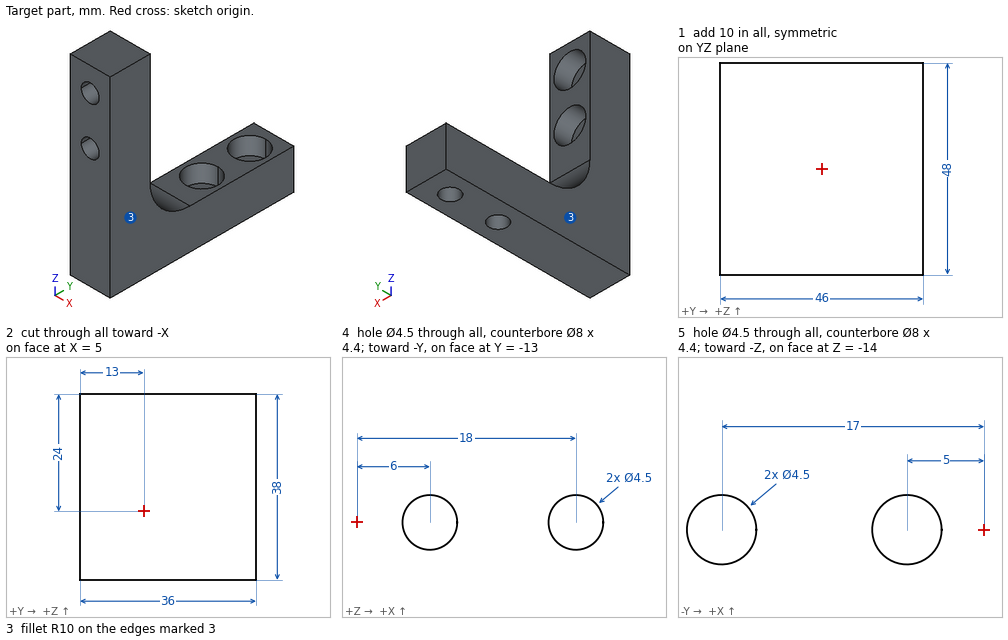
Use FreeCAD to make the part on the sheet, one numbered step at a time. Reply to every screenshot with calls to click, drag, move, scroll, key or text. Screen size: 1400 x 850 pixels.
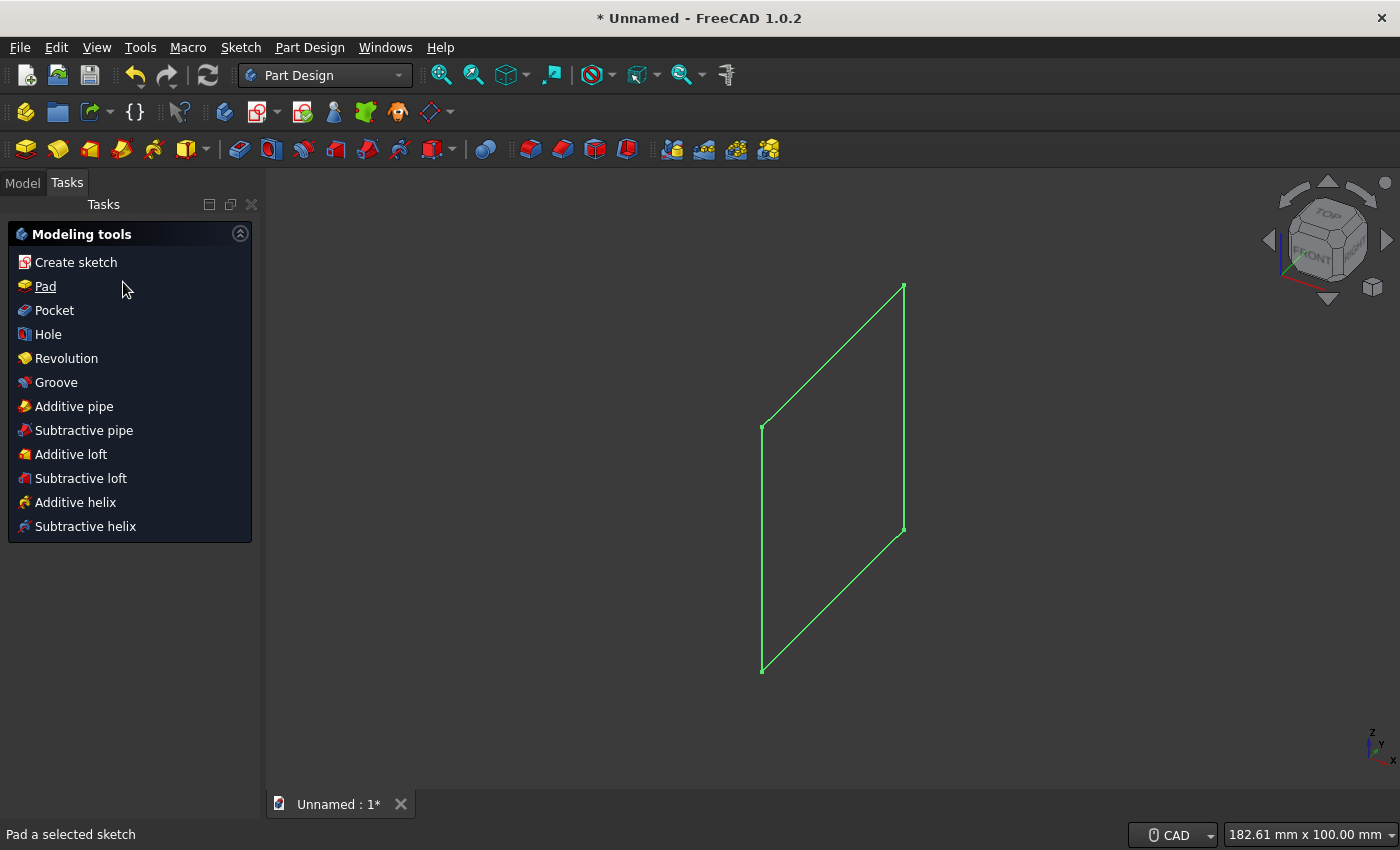
click(26, 150)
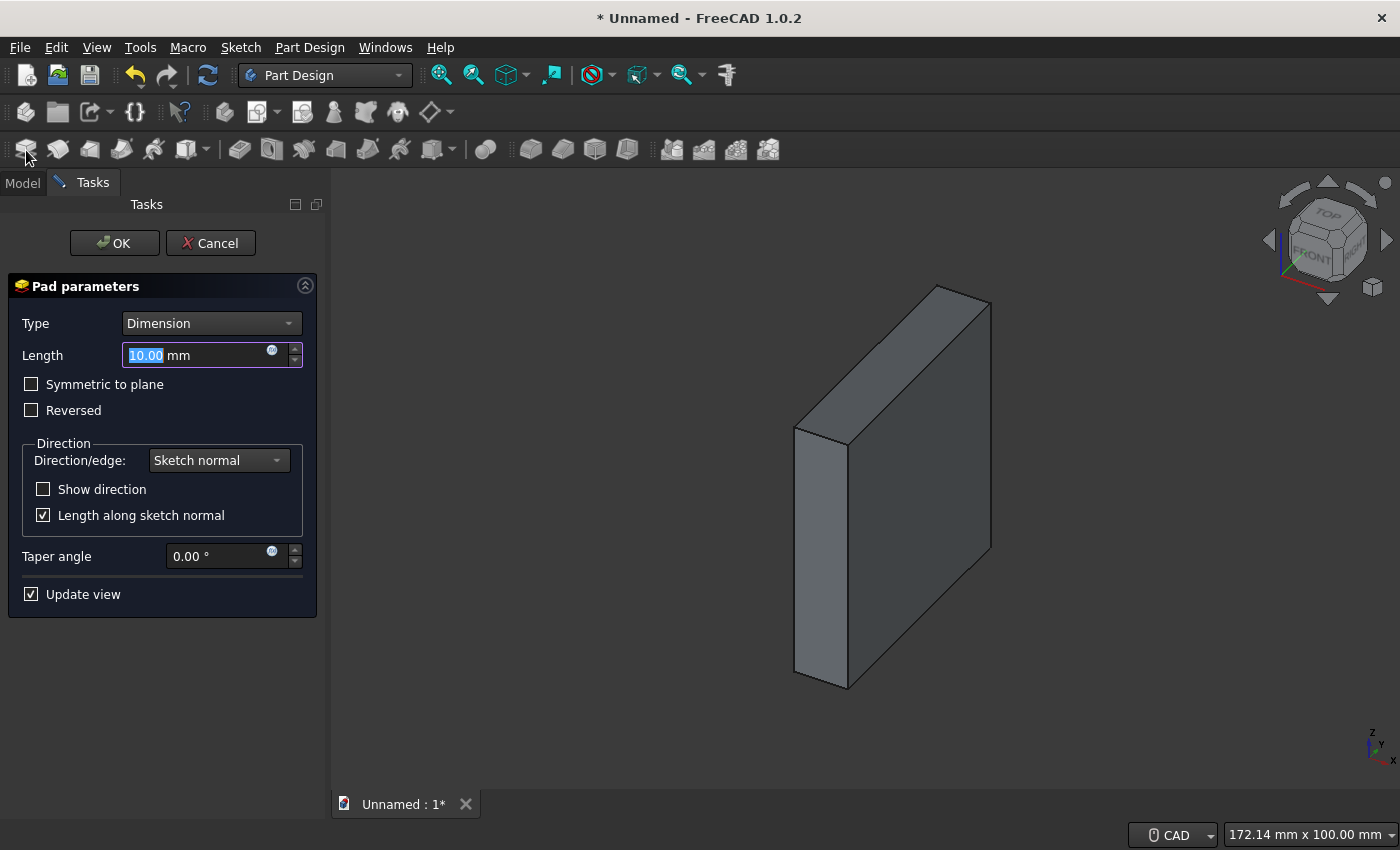
text(10)
key(Tab)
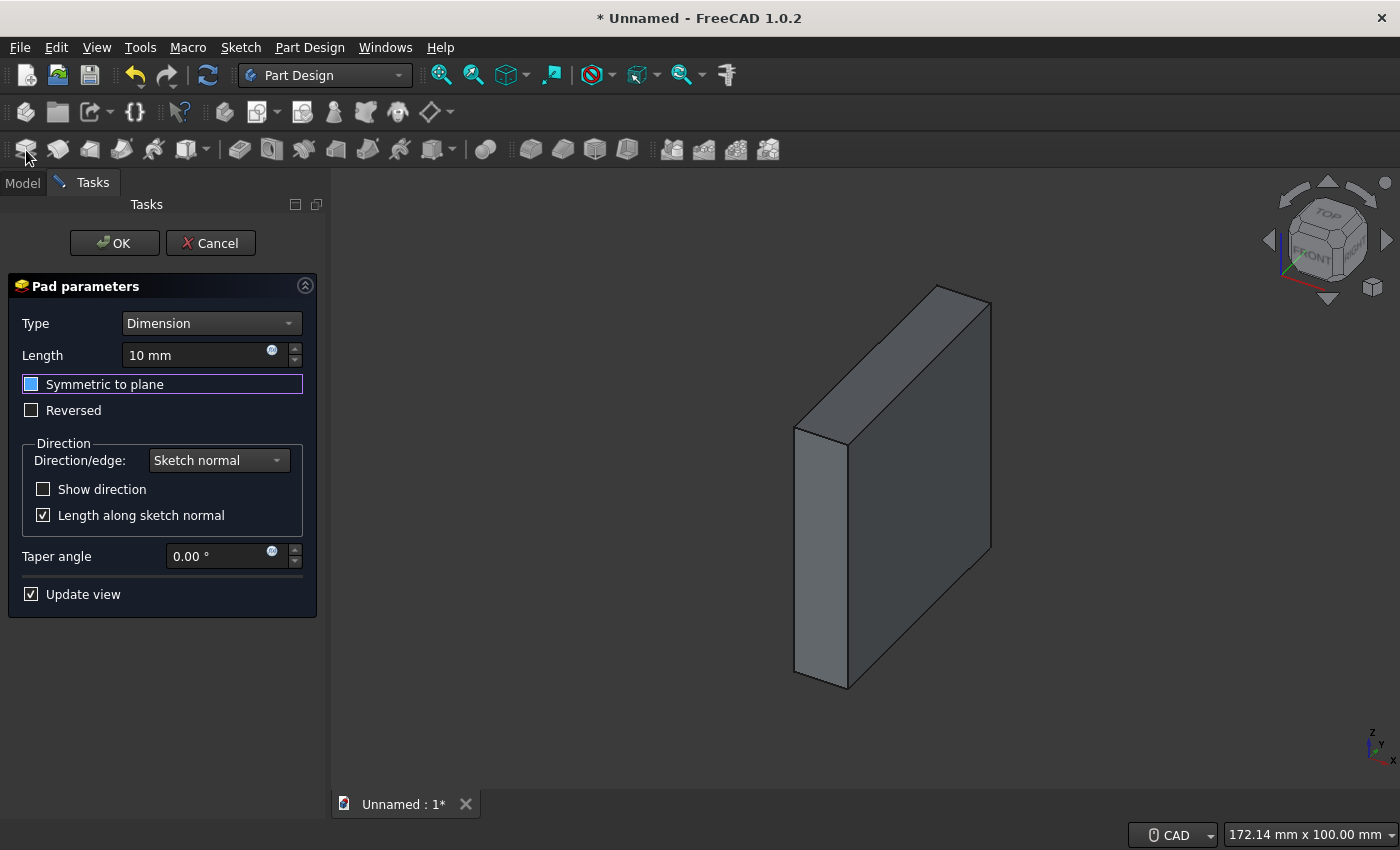
click(30, 384)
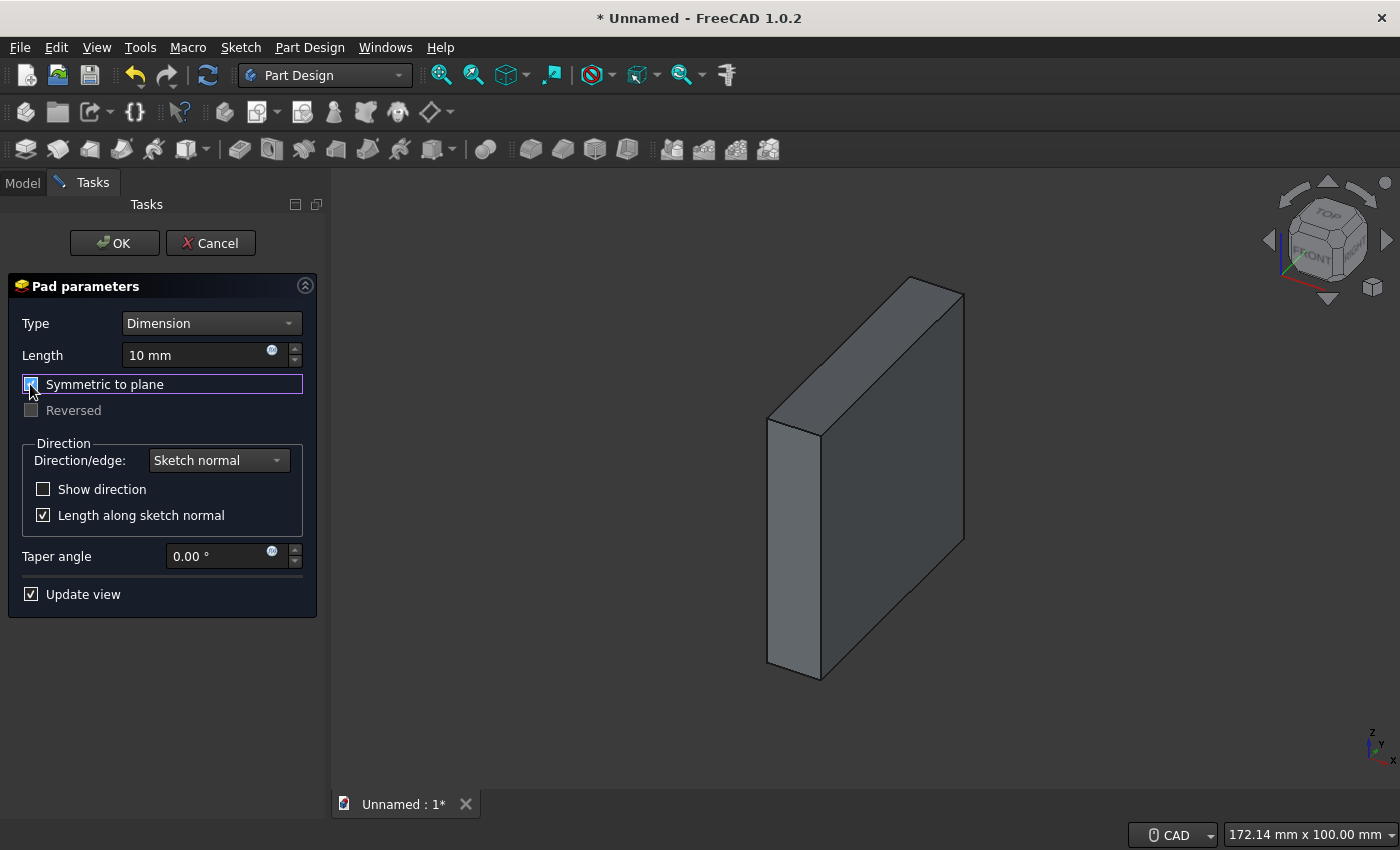
click(115, 243)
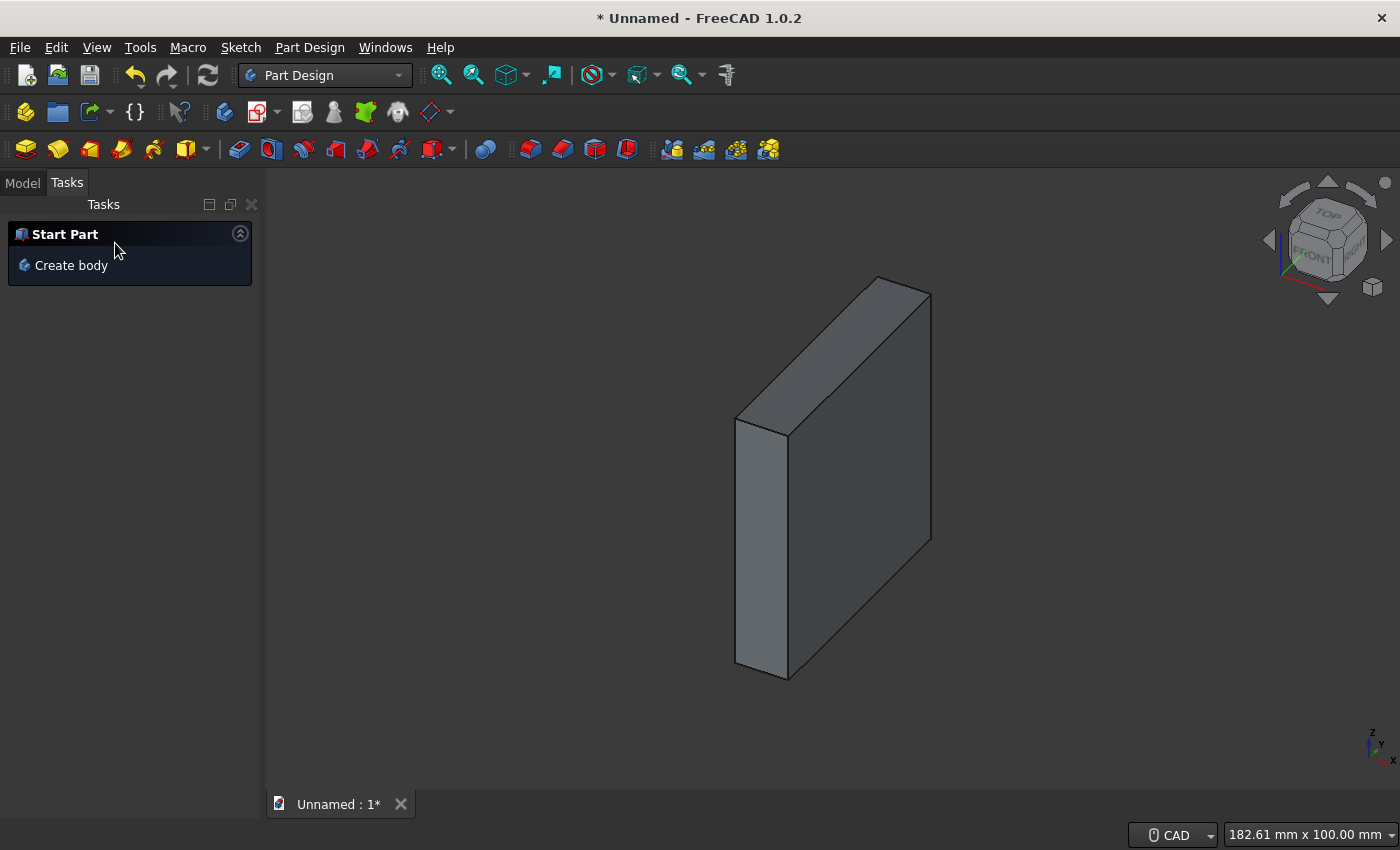
click(860, 486)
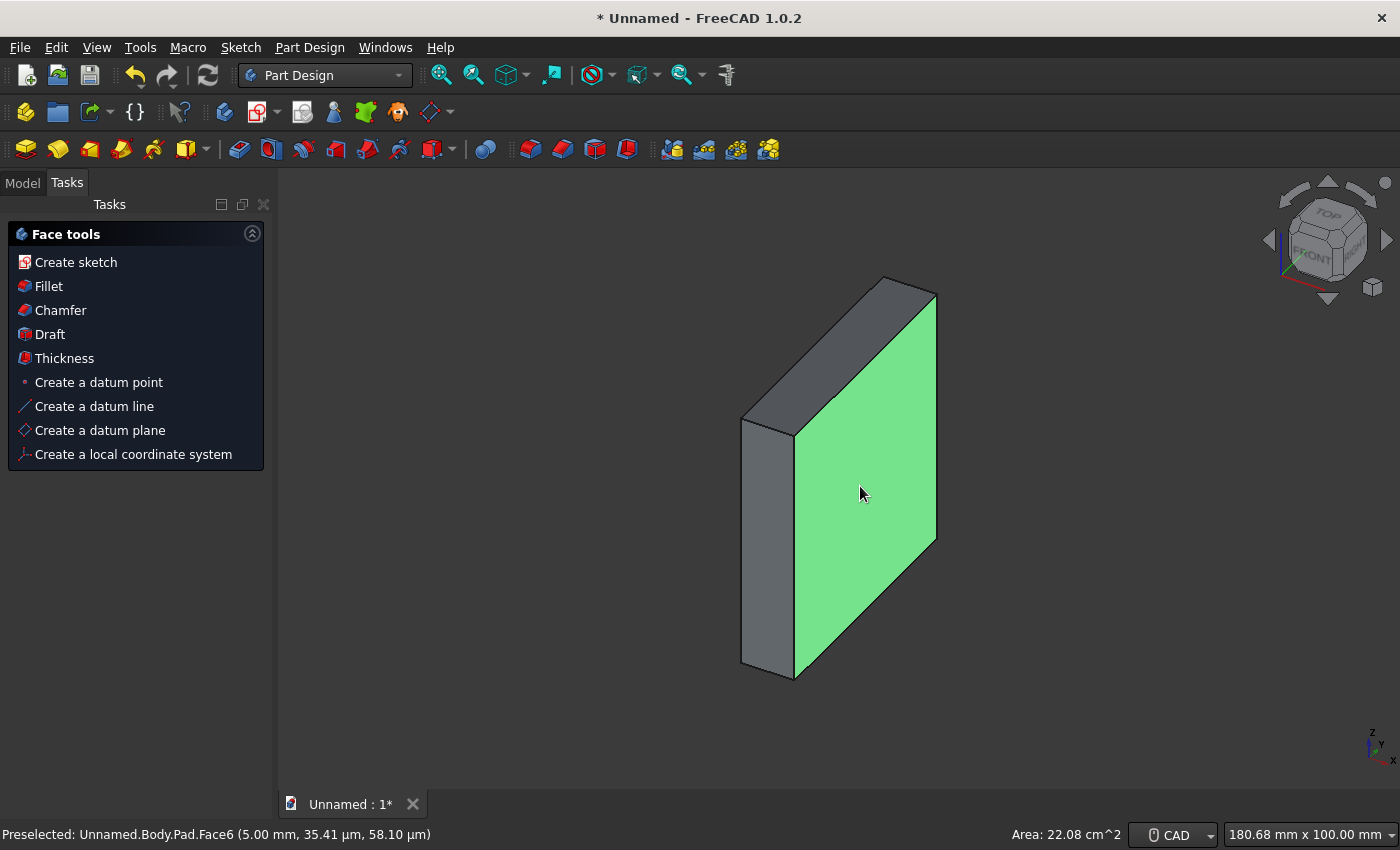
click(258, 112)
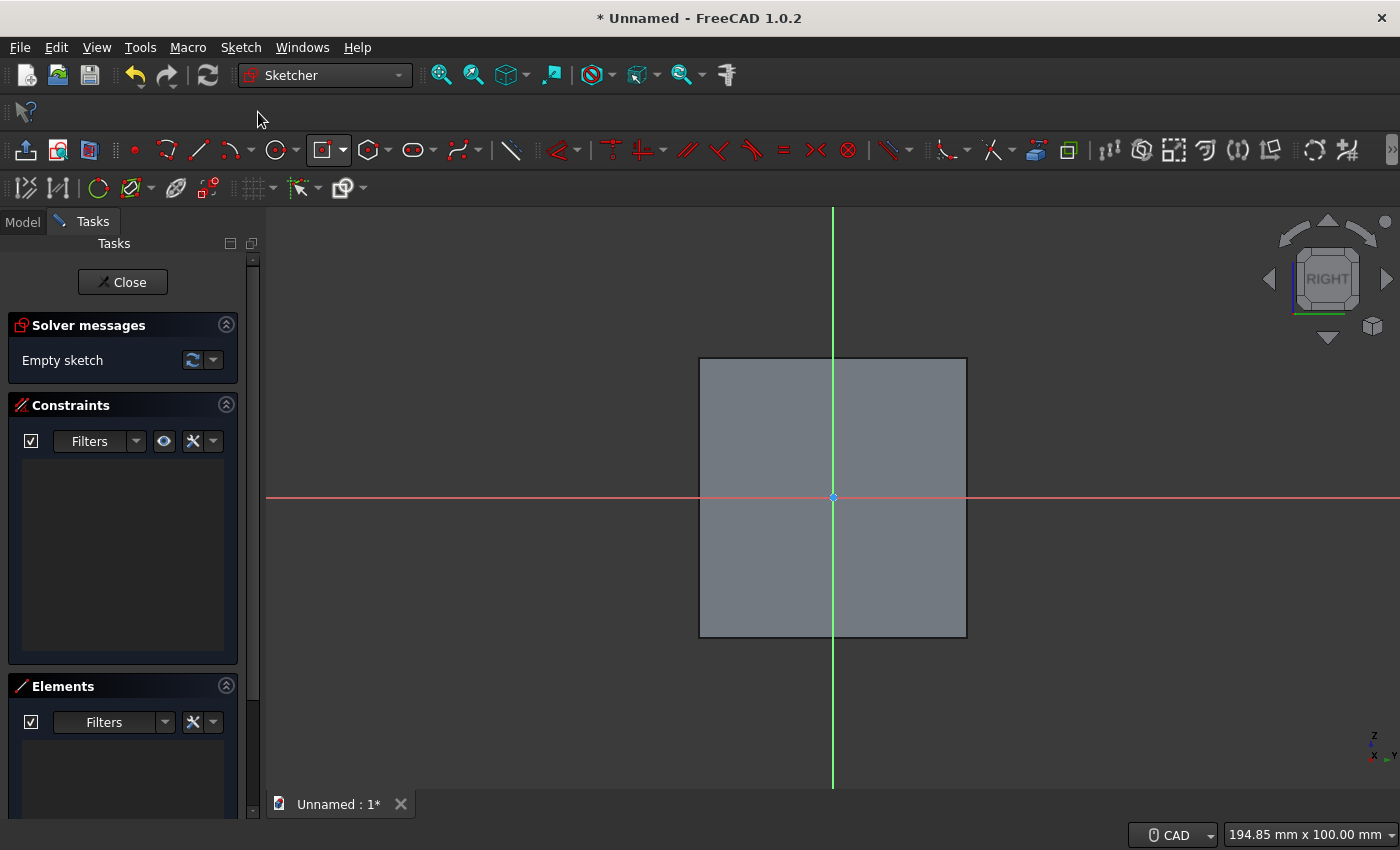
scroll(981, 434, up, 3)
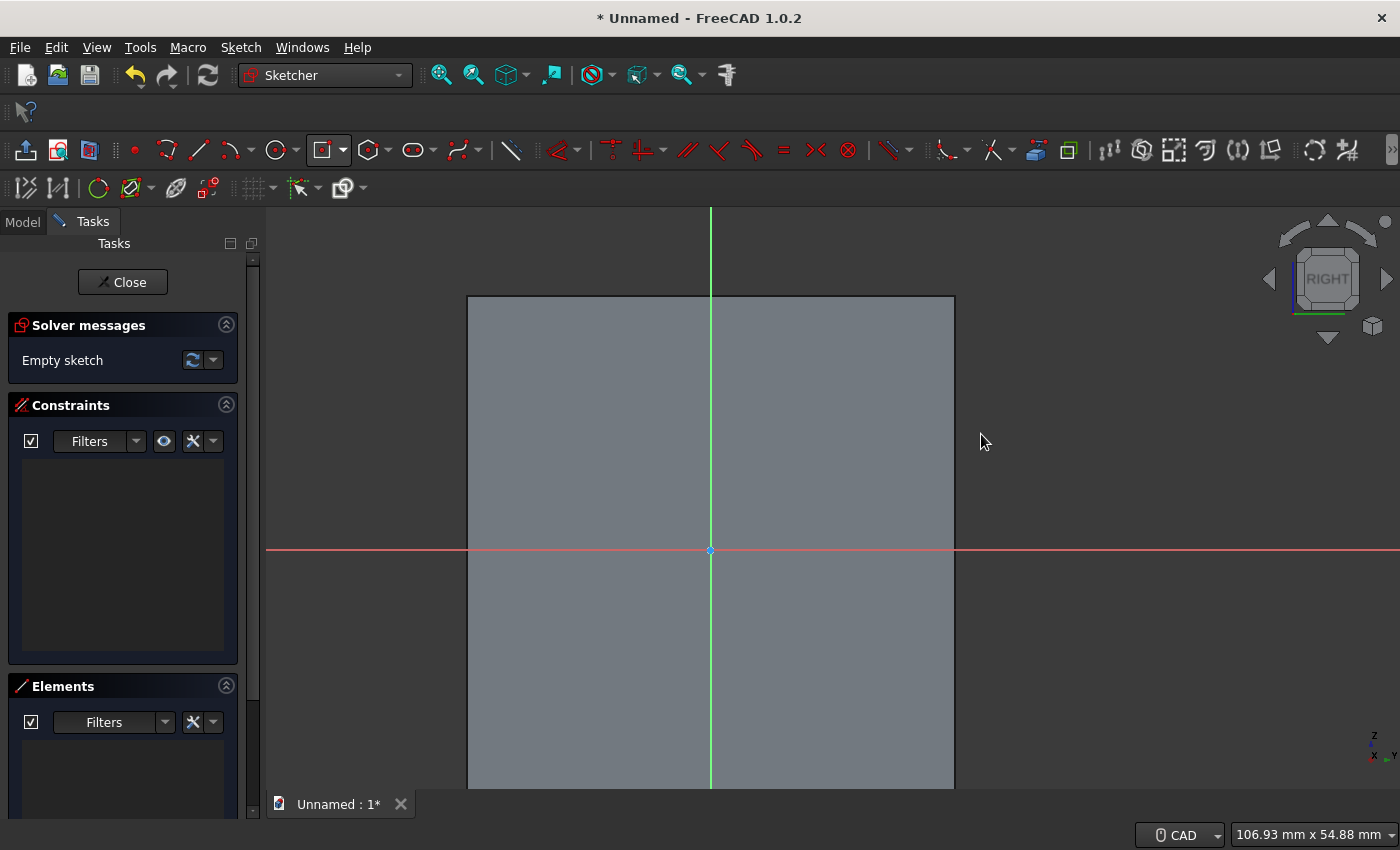
click(346, 150)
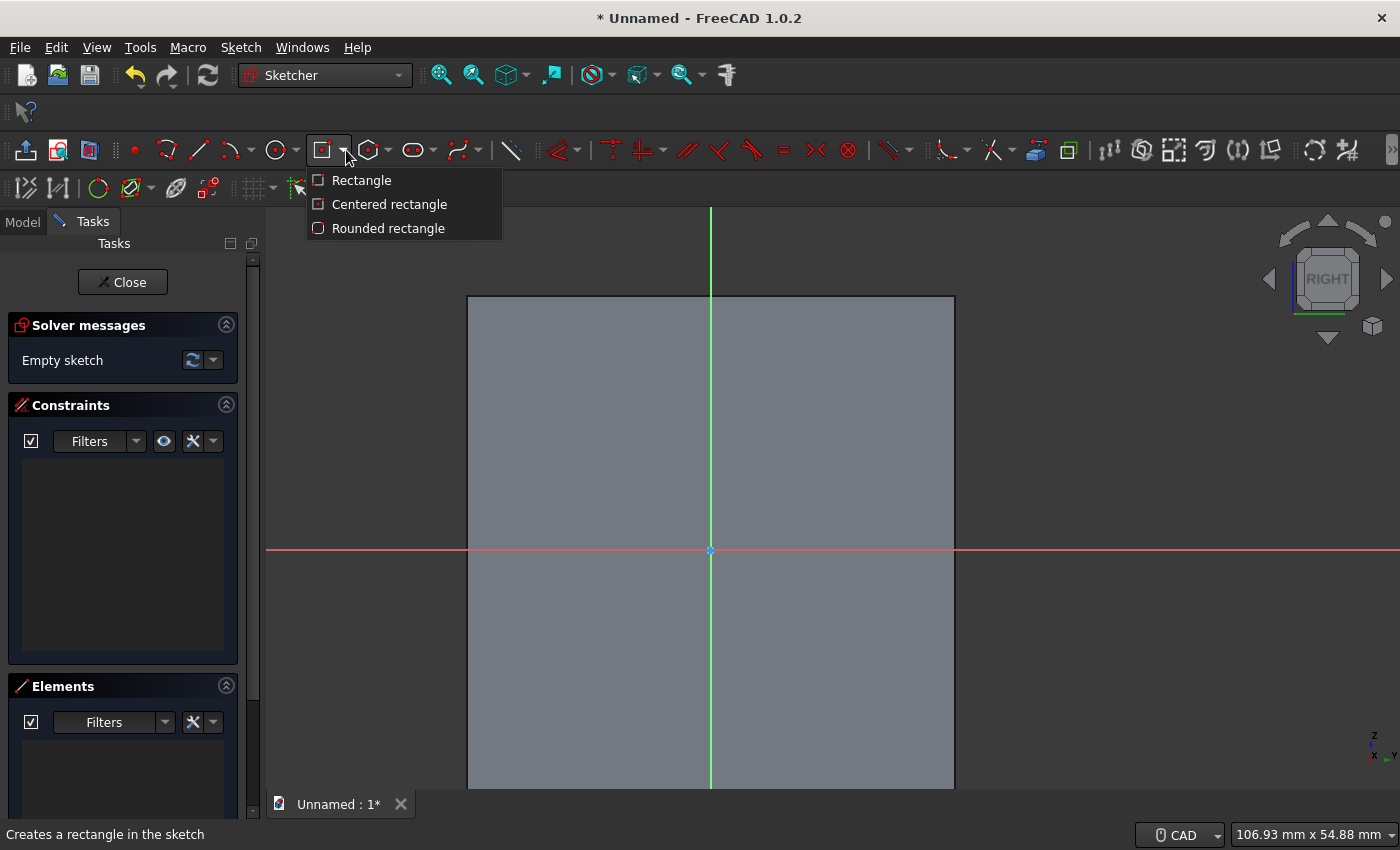
click(404, 180)